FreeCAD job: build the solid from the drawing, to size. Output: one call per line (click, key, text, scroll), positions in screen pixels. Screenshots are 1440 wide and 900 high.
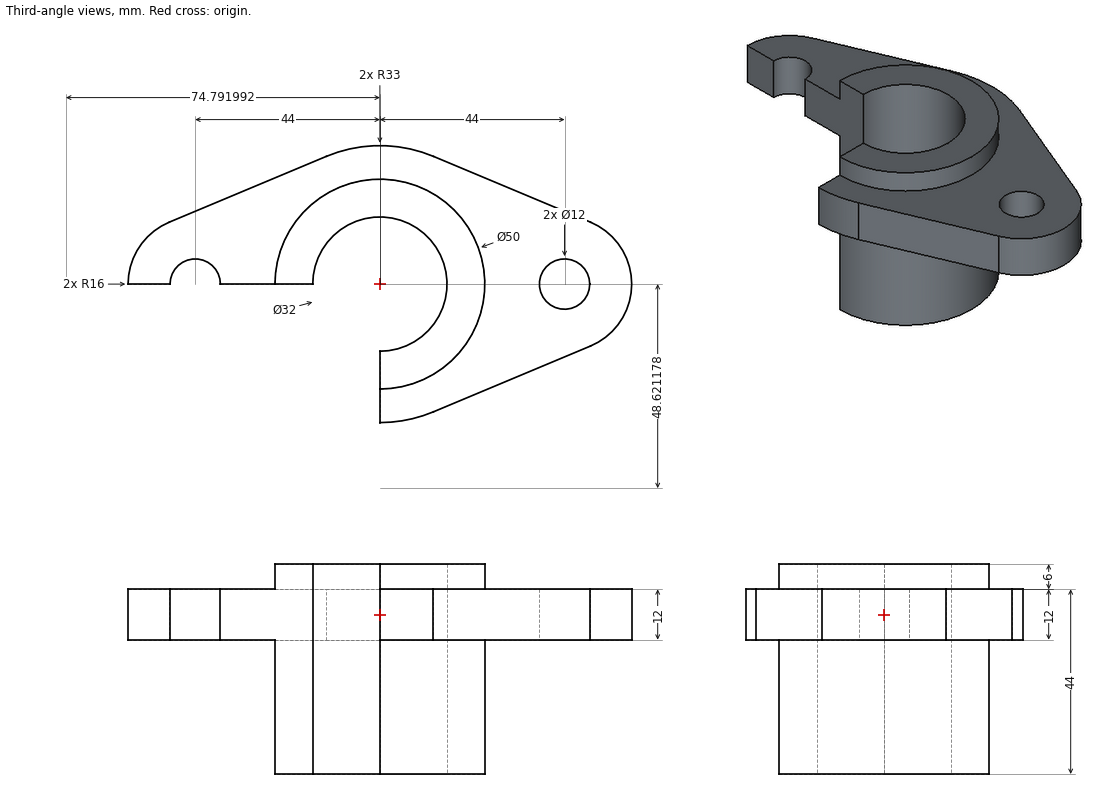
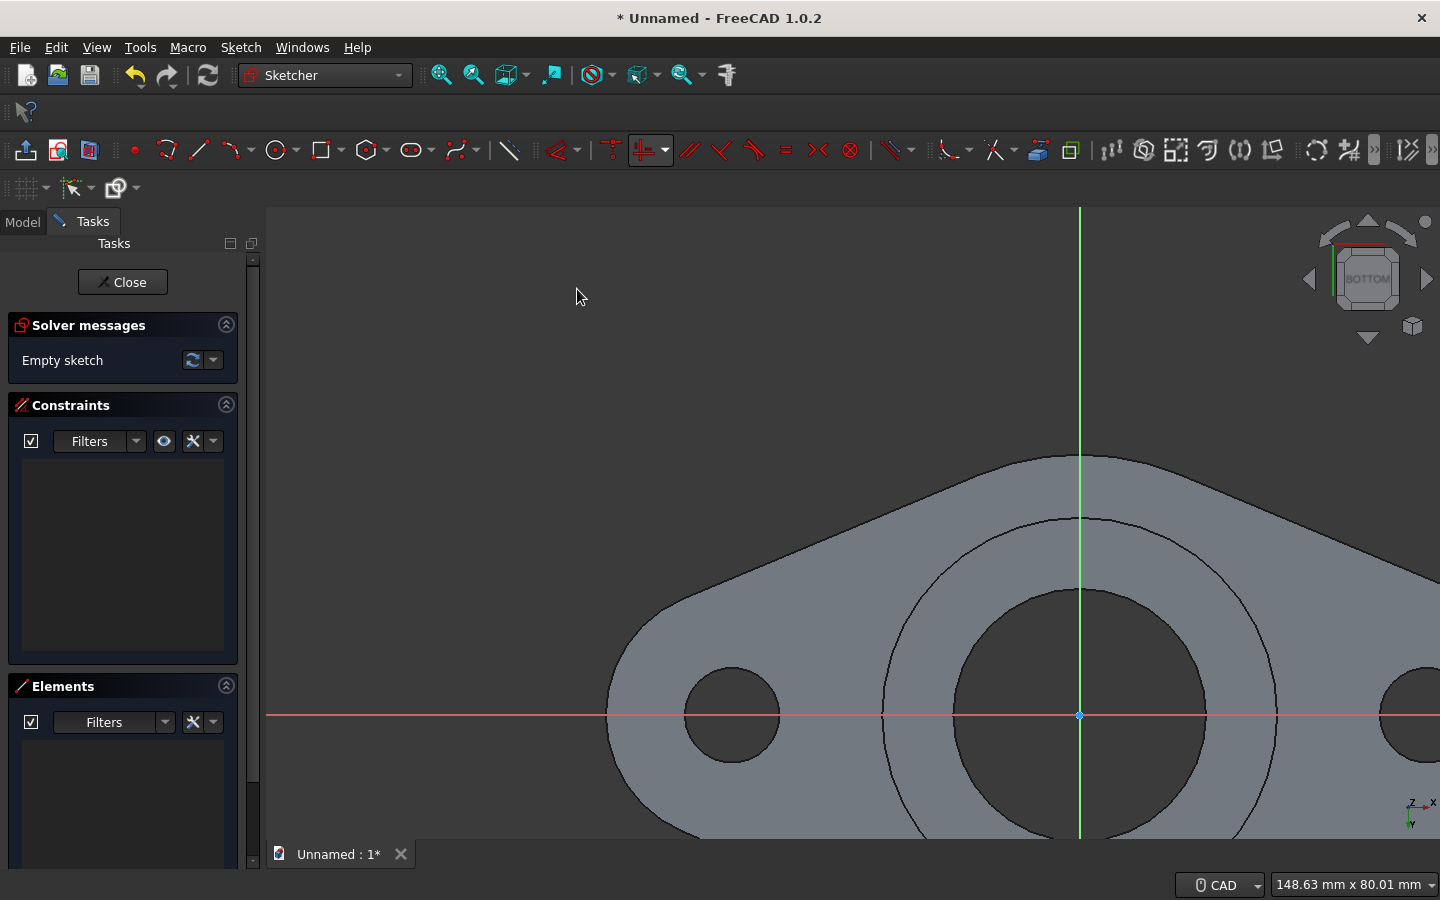
click(168, 150)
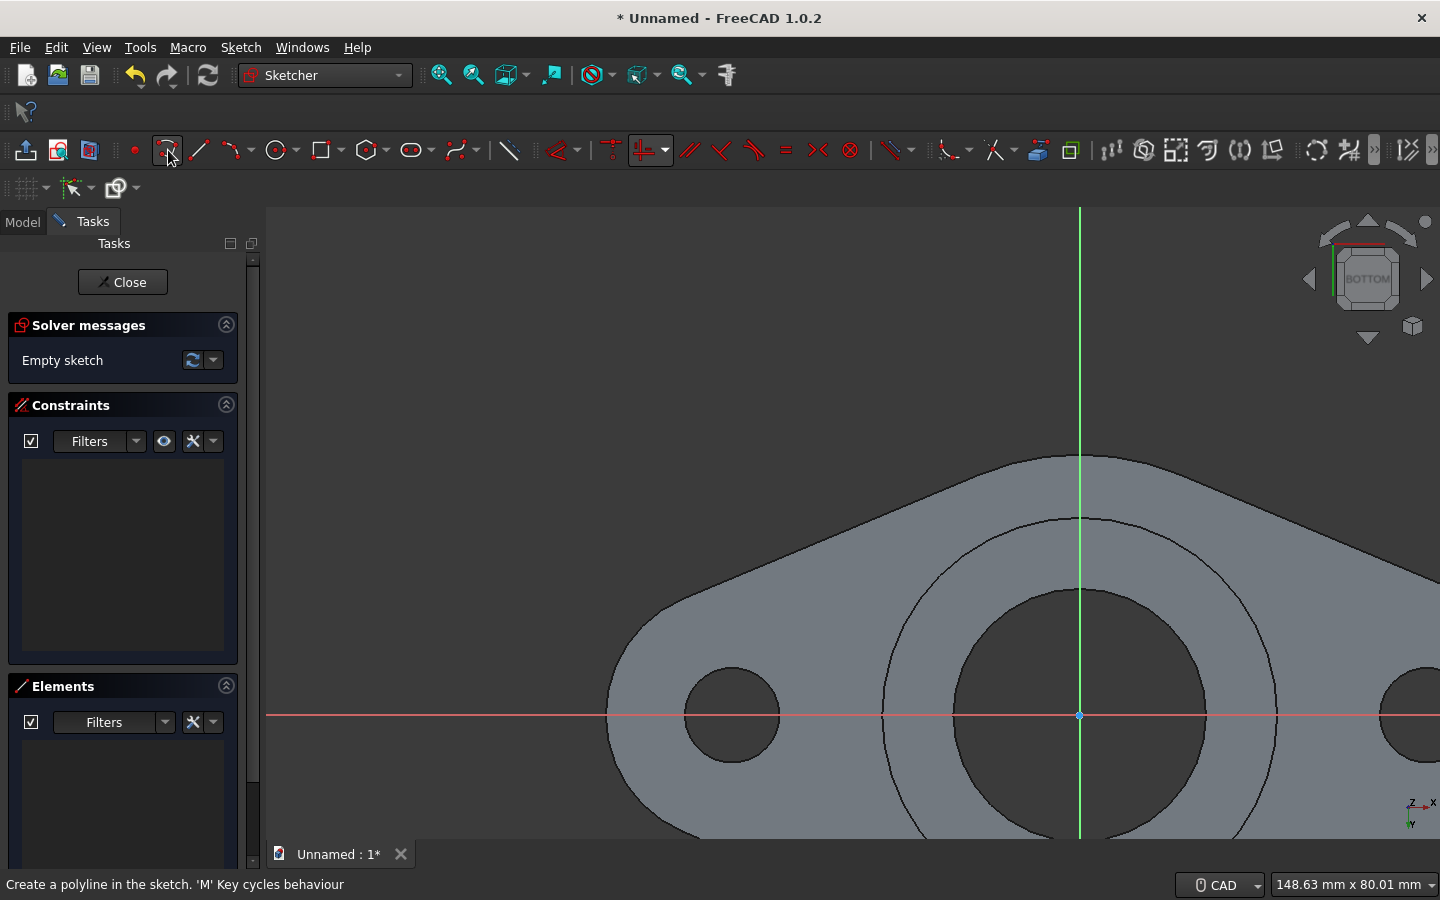
click(1080, 715)
click(1071, 331)
click(489, 706)
click(1080, 715)
key(Escape)
key(Escape)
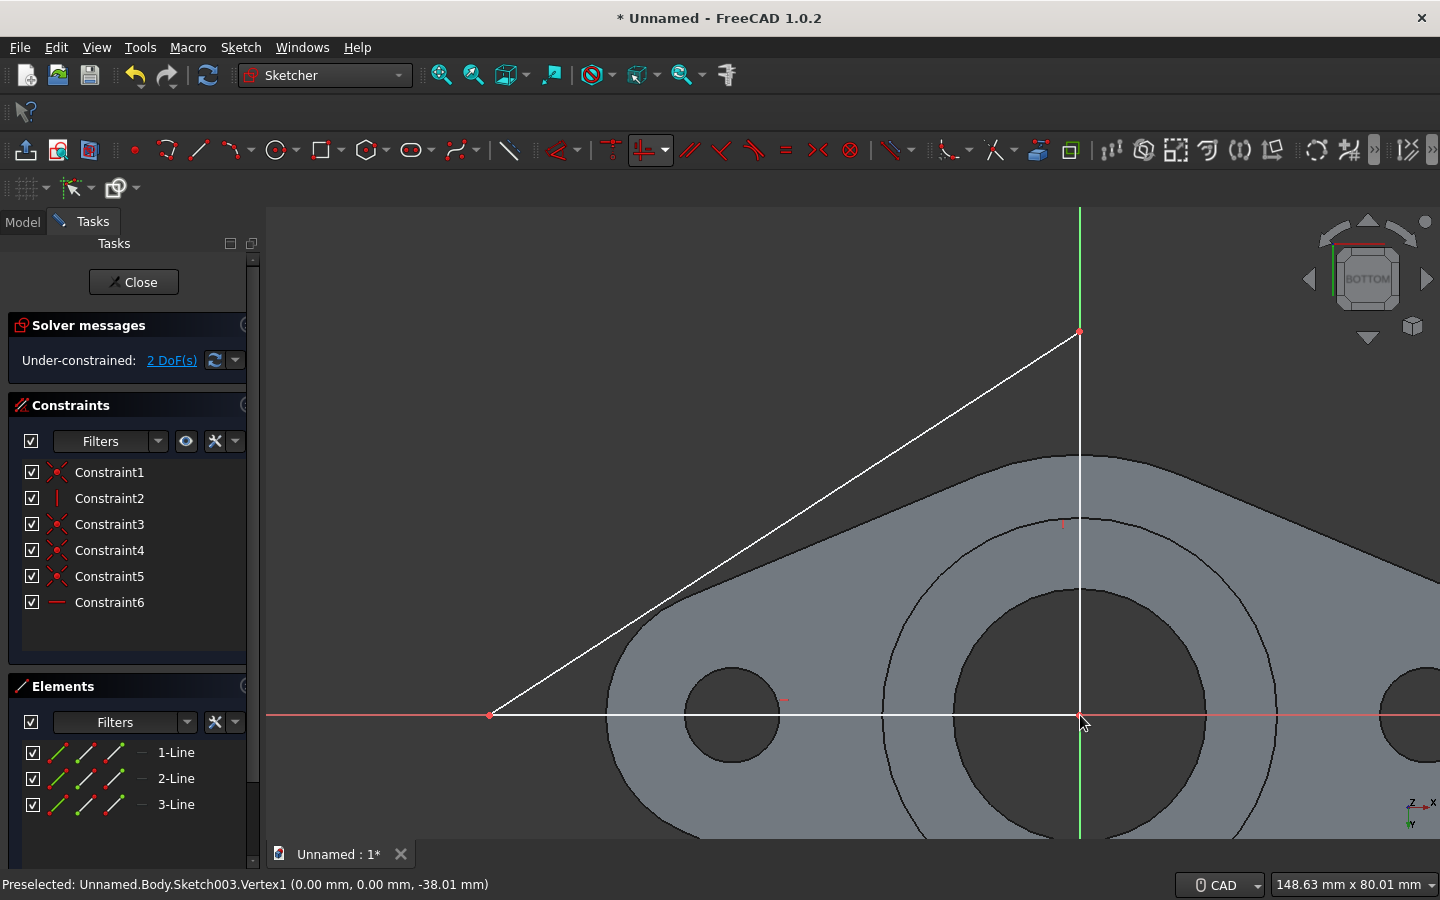
click(556, 150)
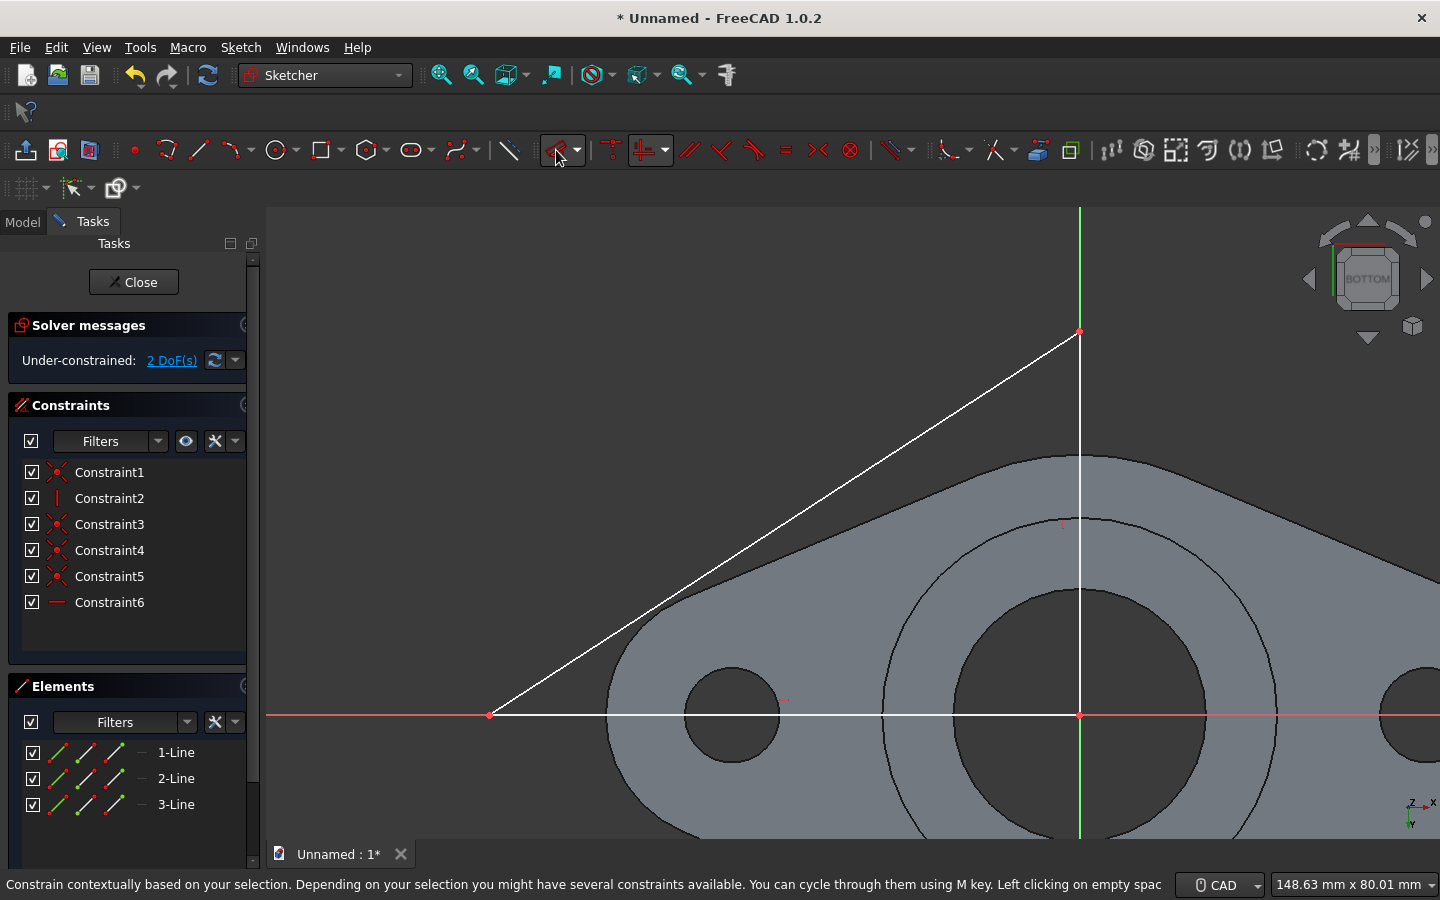
click(1080, 600)
click(1114, 524)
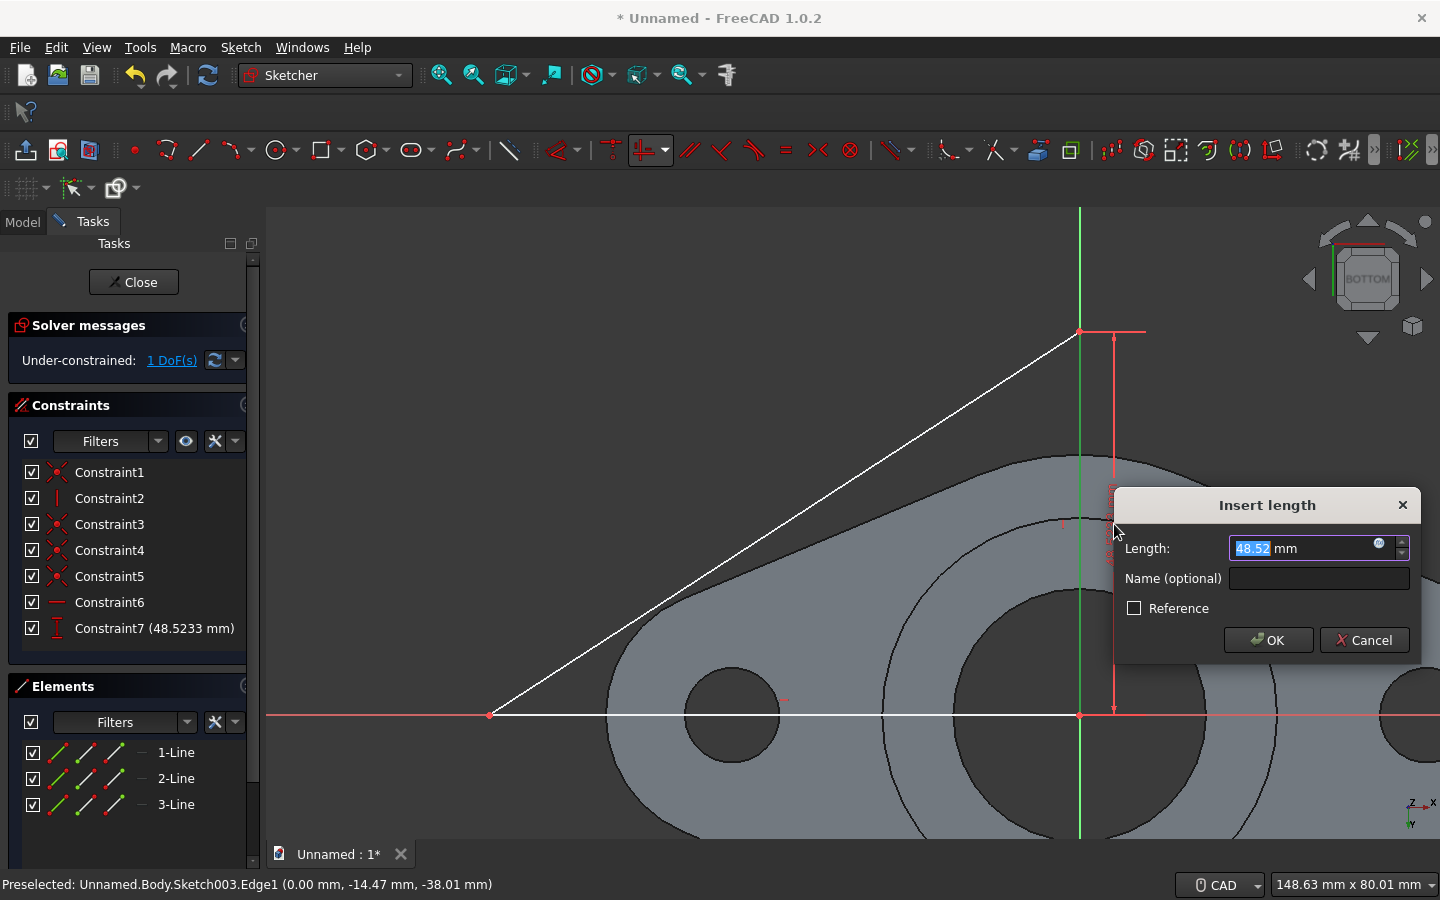
text(48.621178)
key(Return)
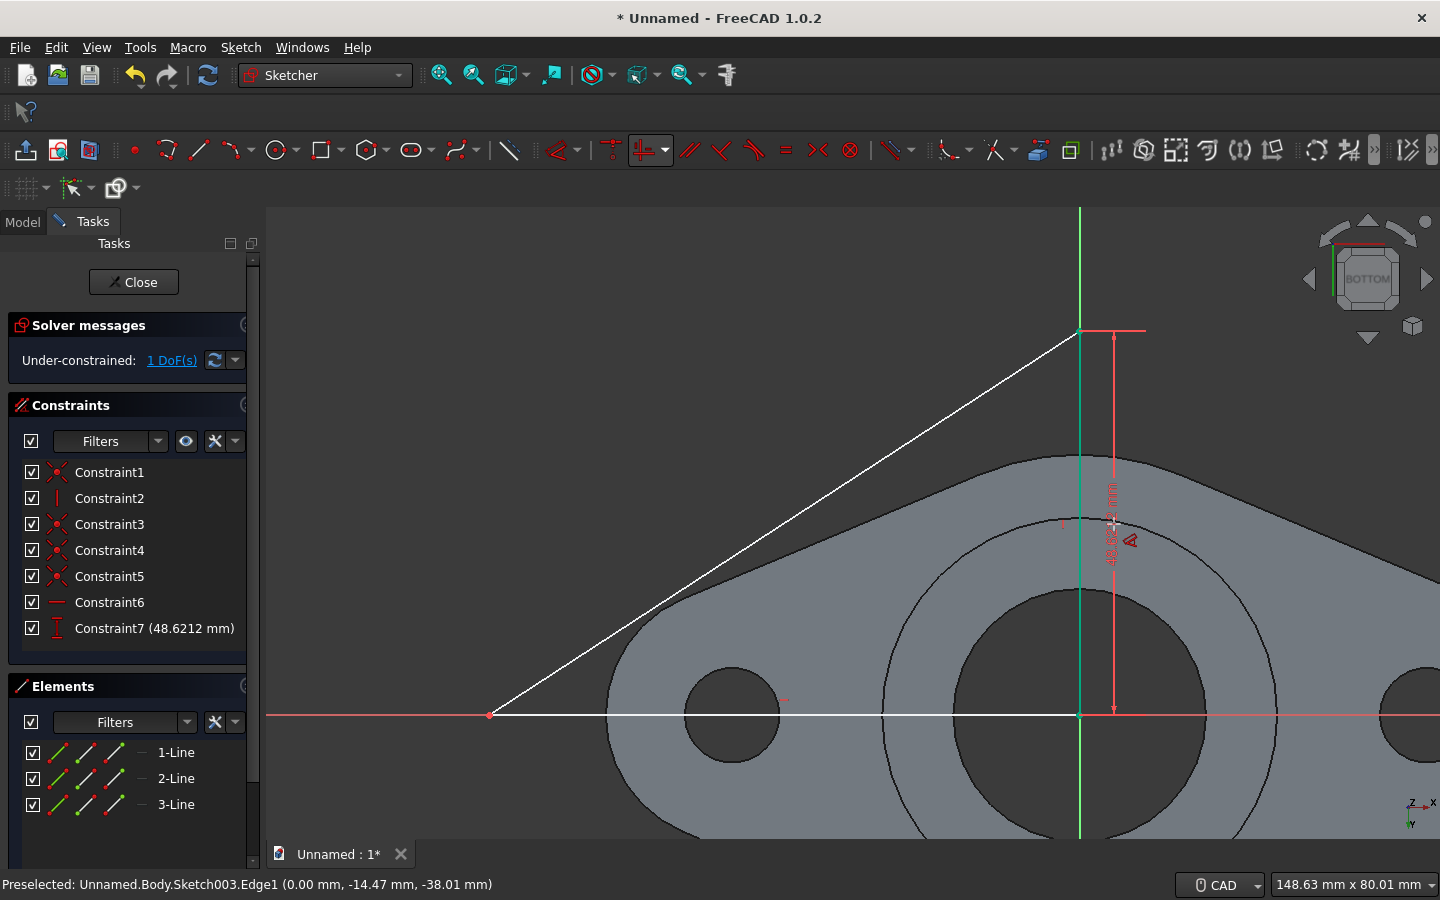
click(666, 715)
click(784, 749)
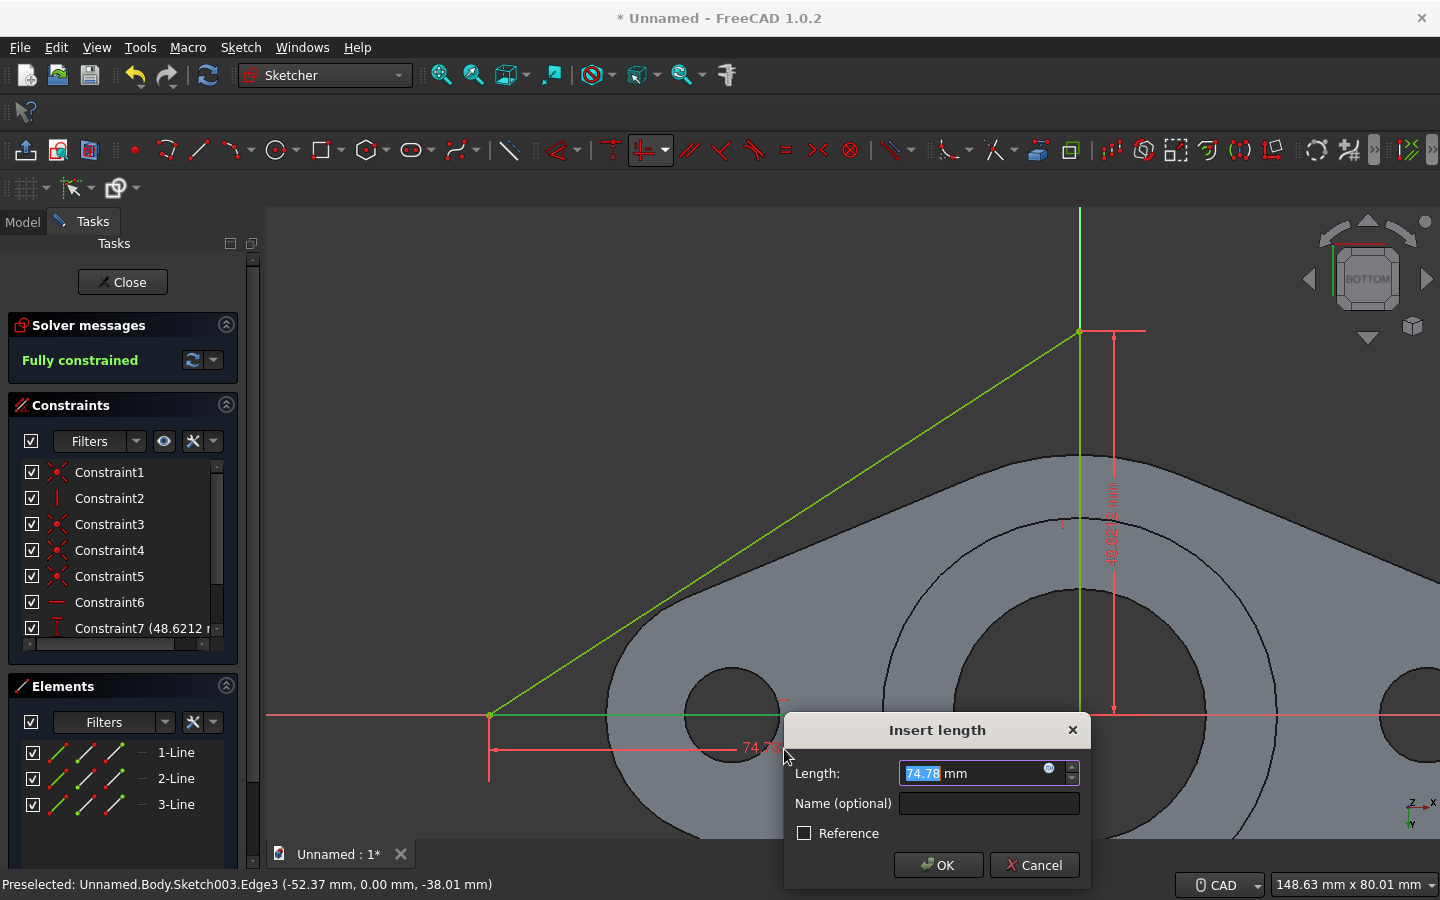
text(74.791992)
key(Return)
key(Escape)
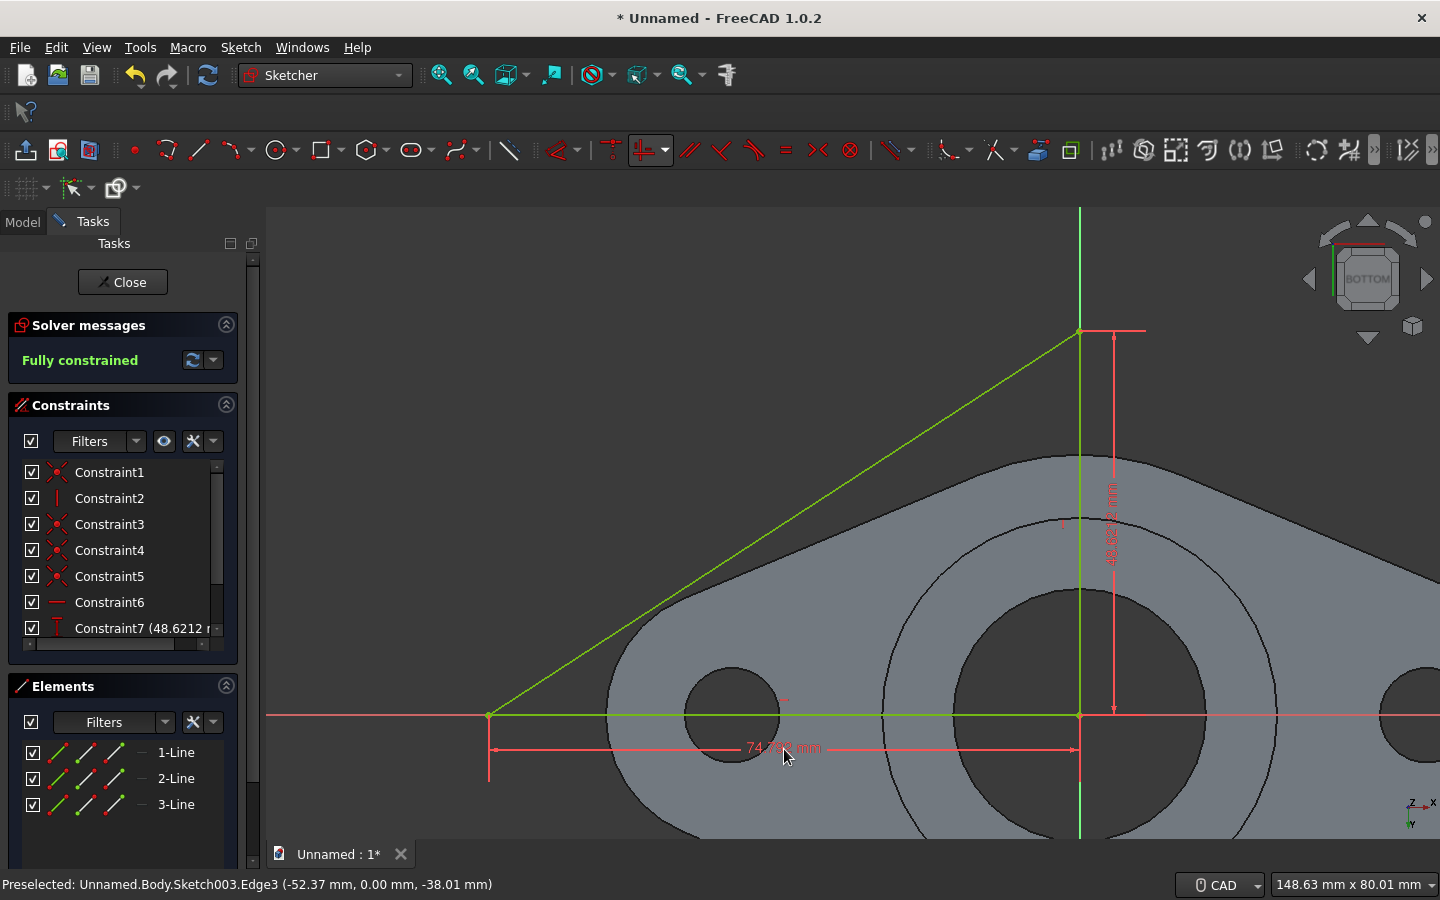
click(123, 282)